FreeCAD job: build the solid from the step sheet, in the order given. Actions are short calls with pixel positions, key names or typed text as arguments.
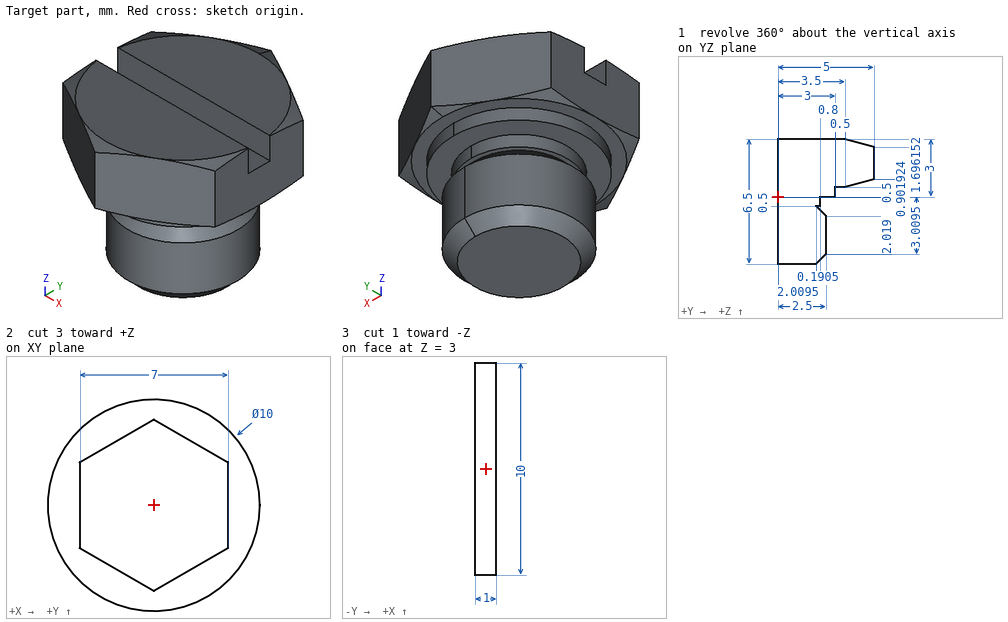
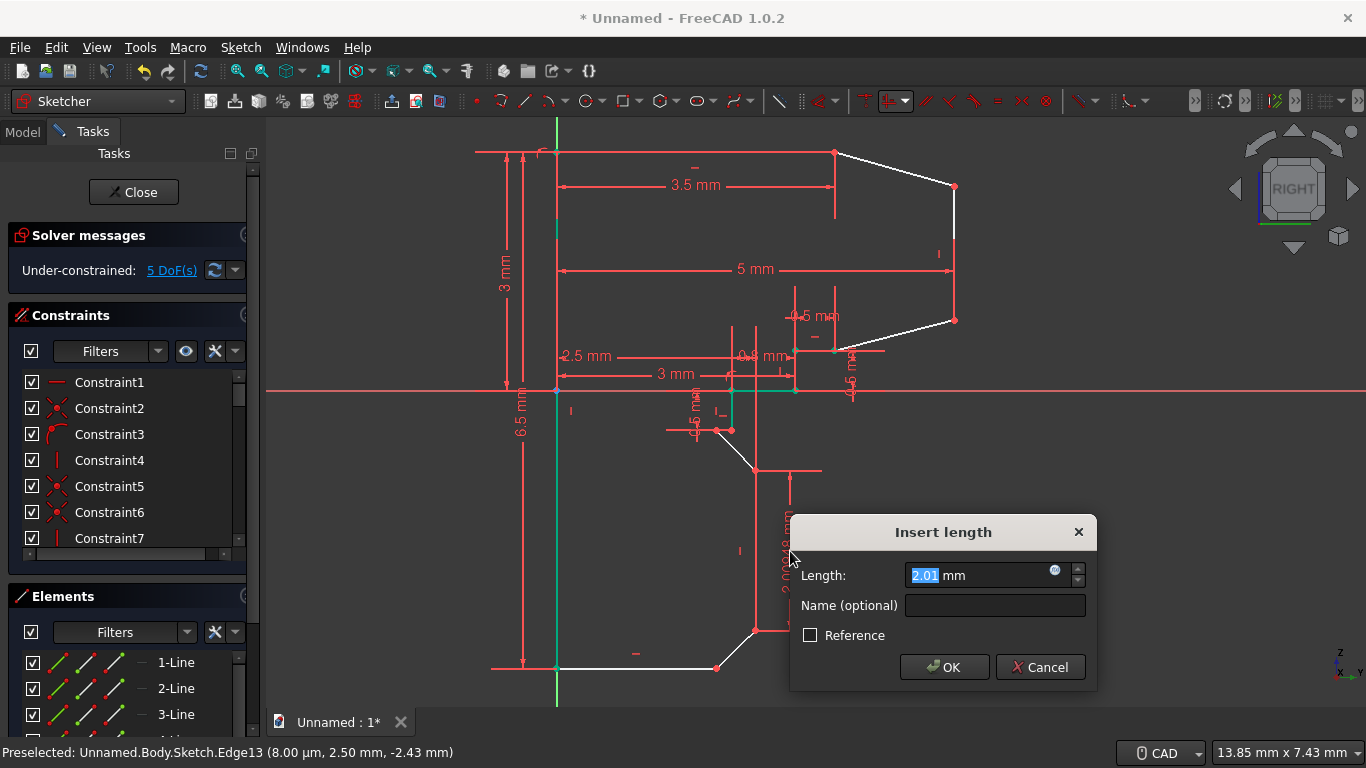
text(2.019)
key(Return)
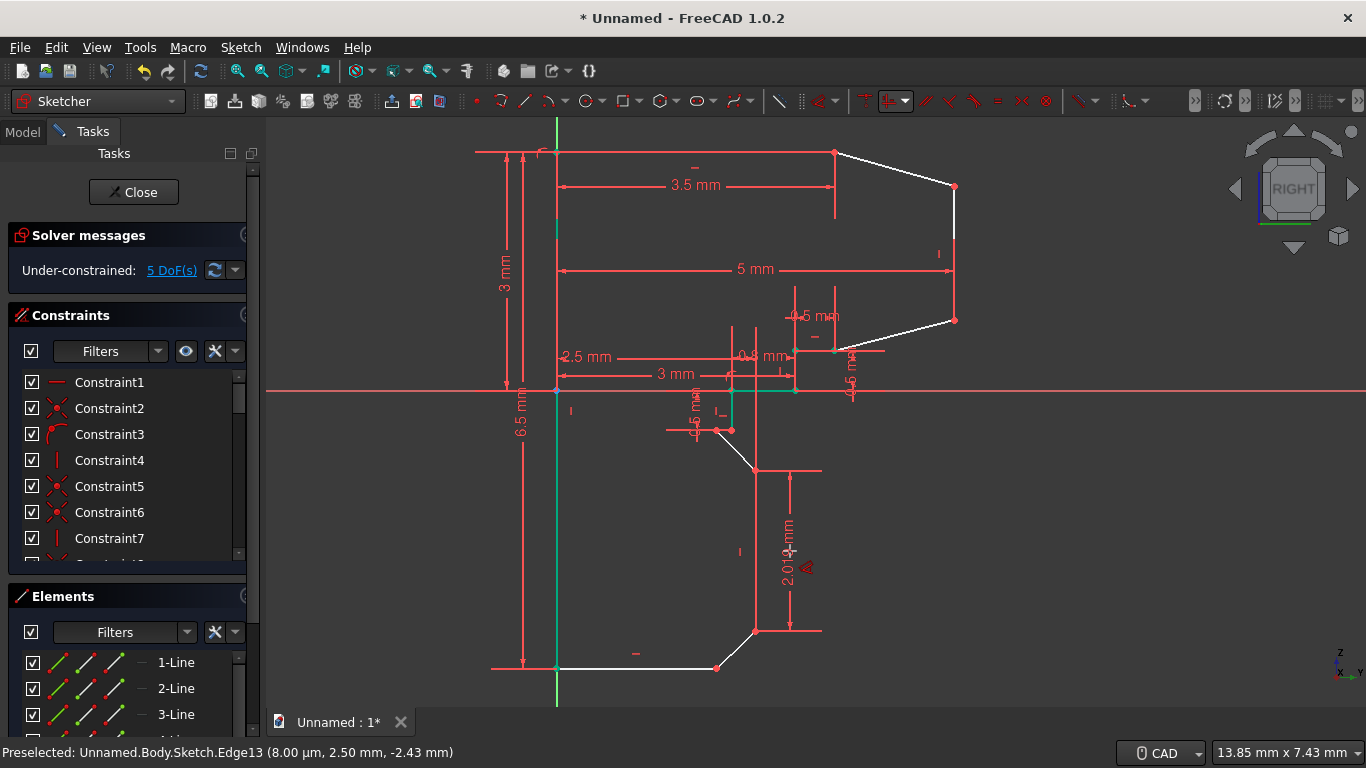
scroll(726, 430, up, 5)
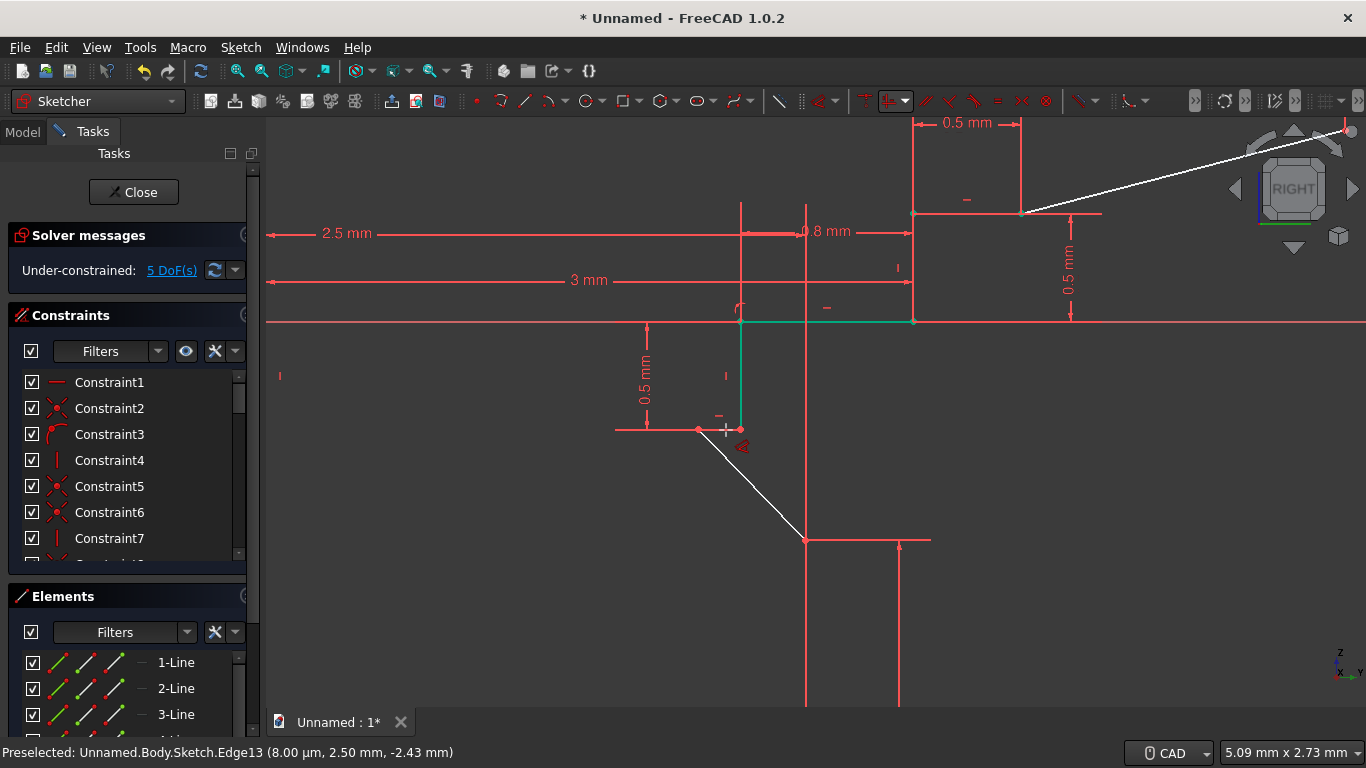
click(724, 430)
click(710, 464)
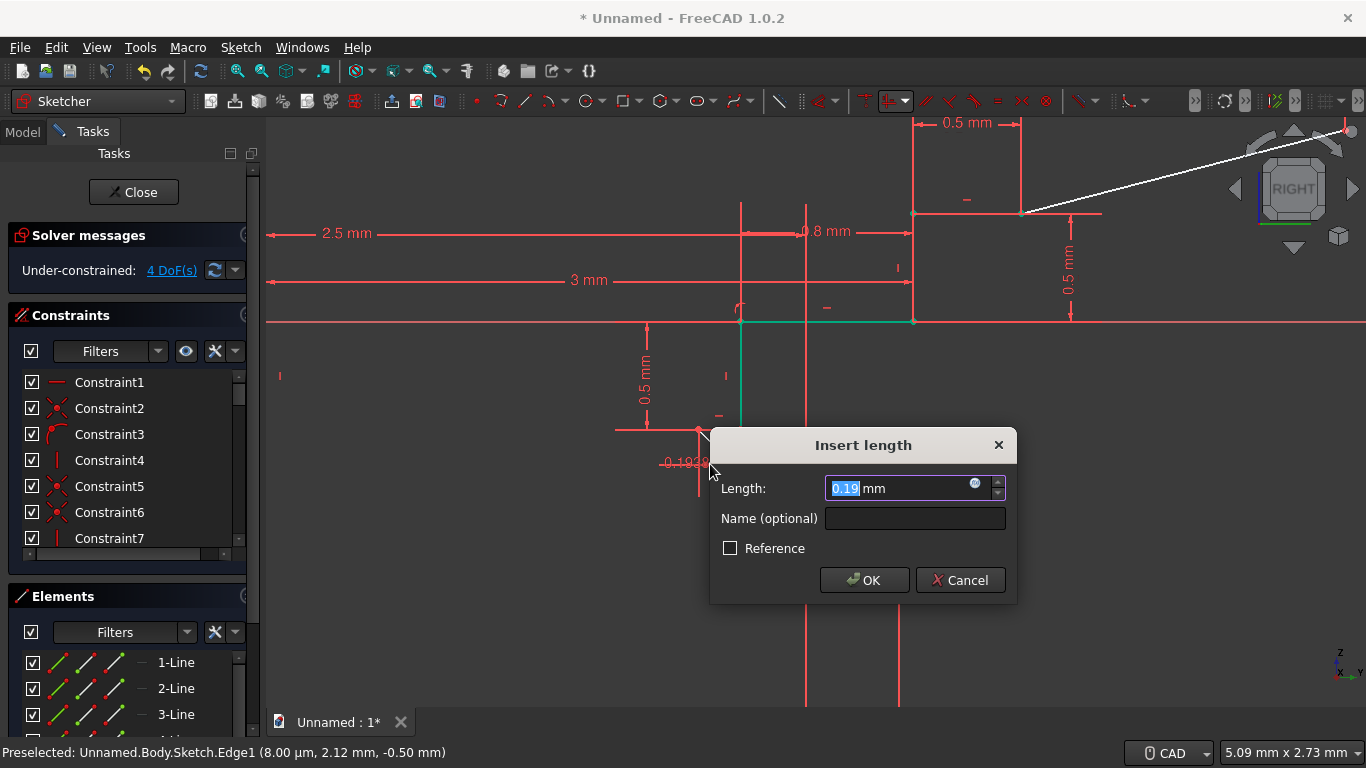
text(0.1905)
key(Return)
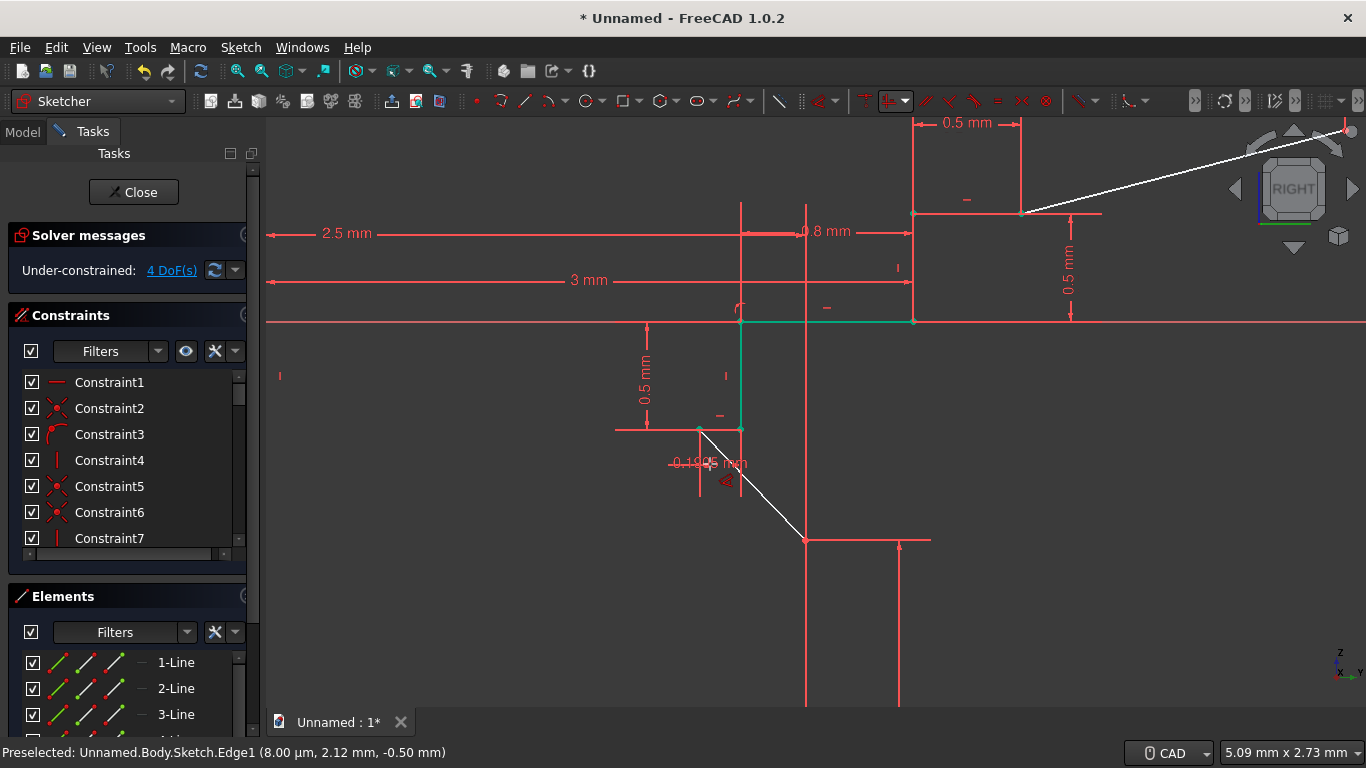
scroll(729, 424, down, 7)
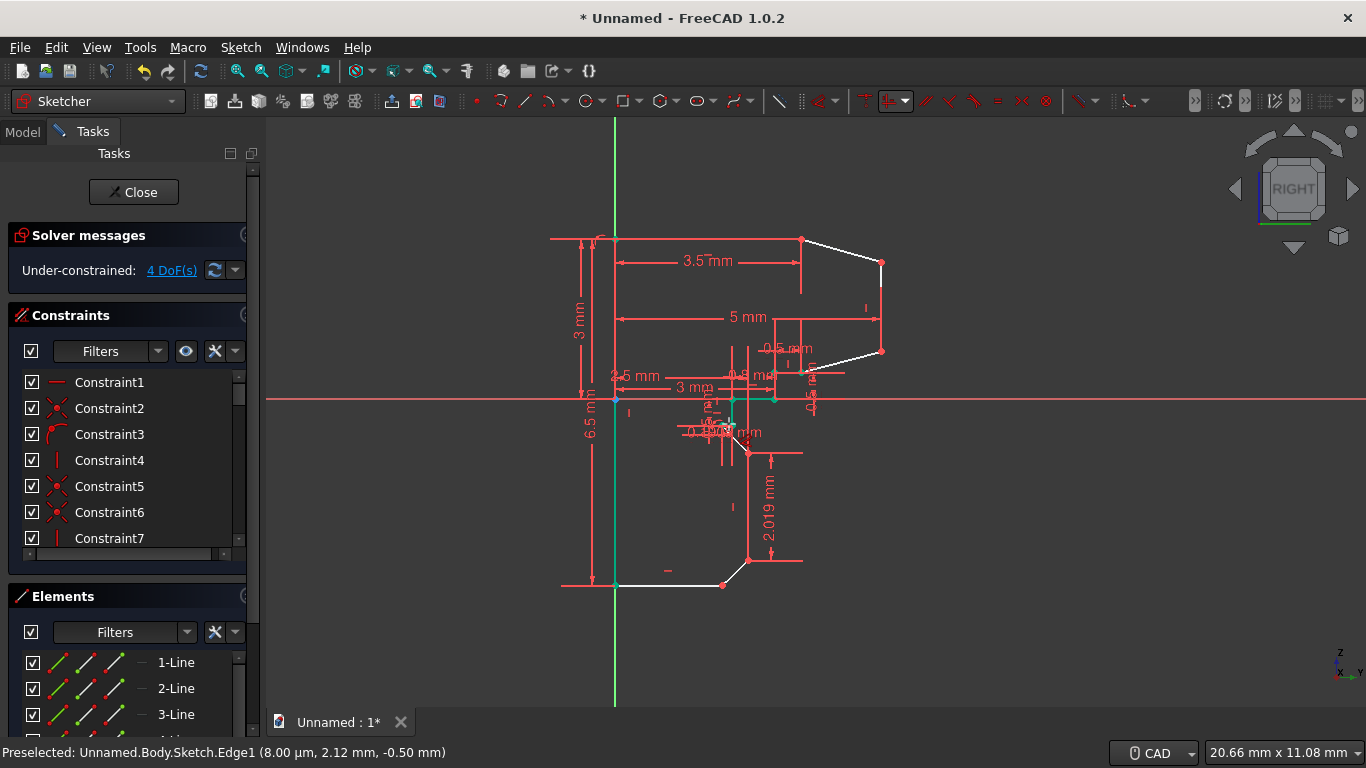
click(647, 586)
click(669, 620)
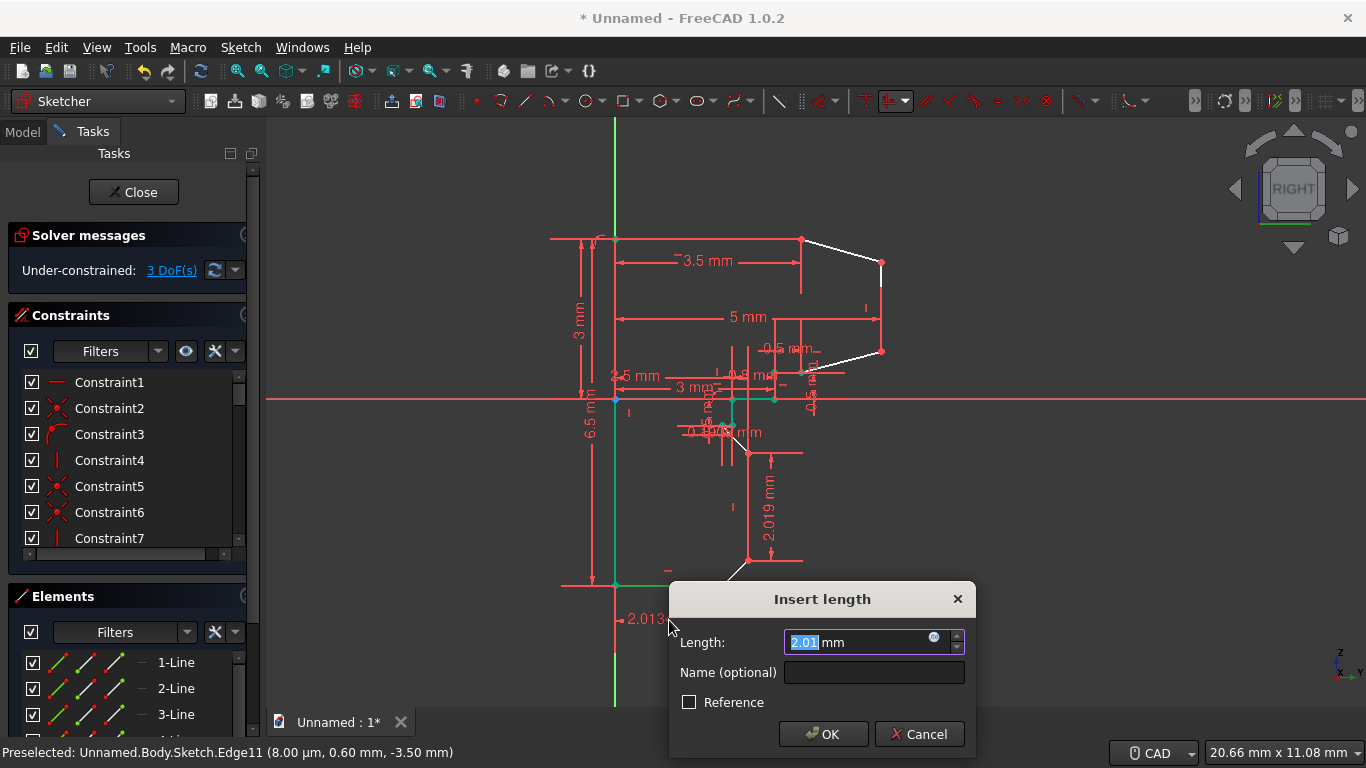
text(2.0095)
key(Return)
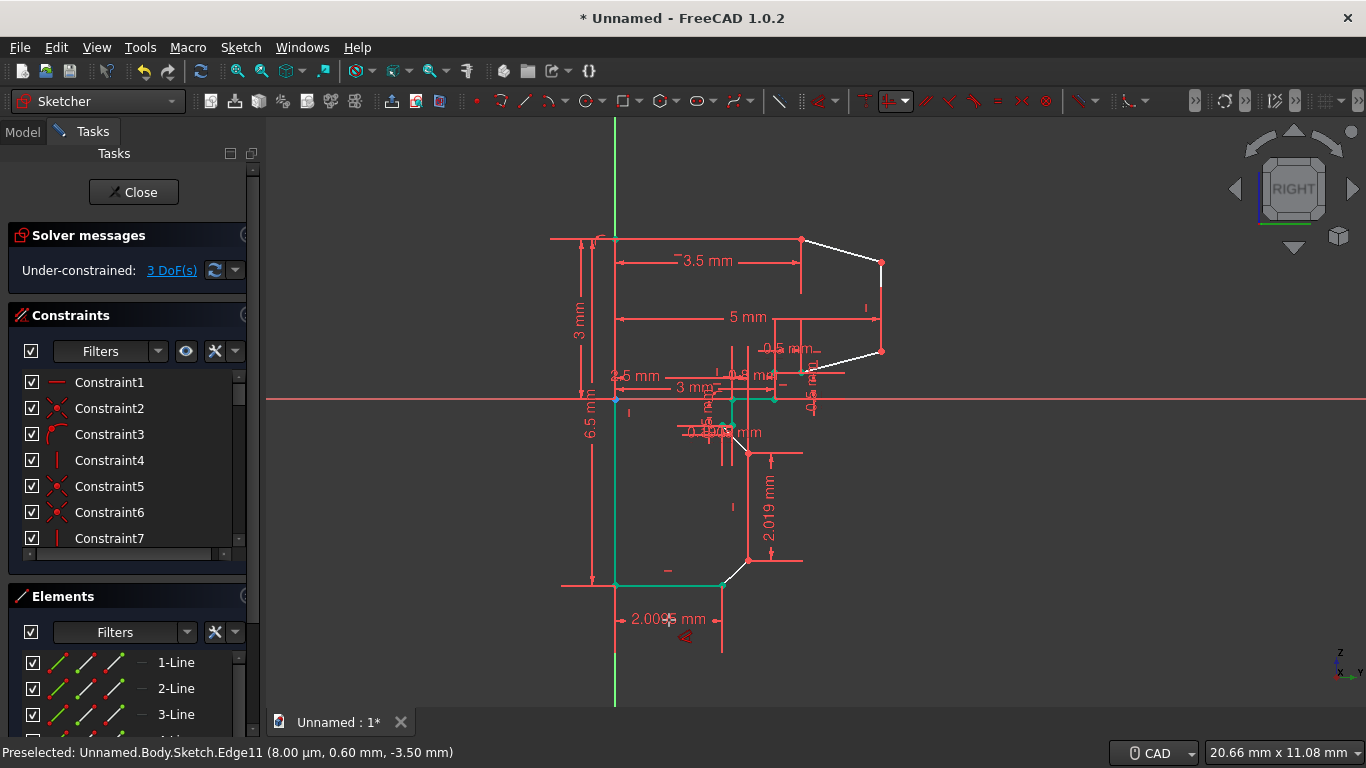
click(748, 561)
click(581, 480)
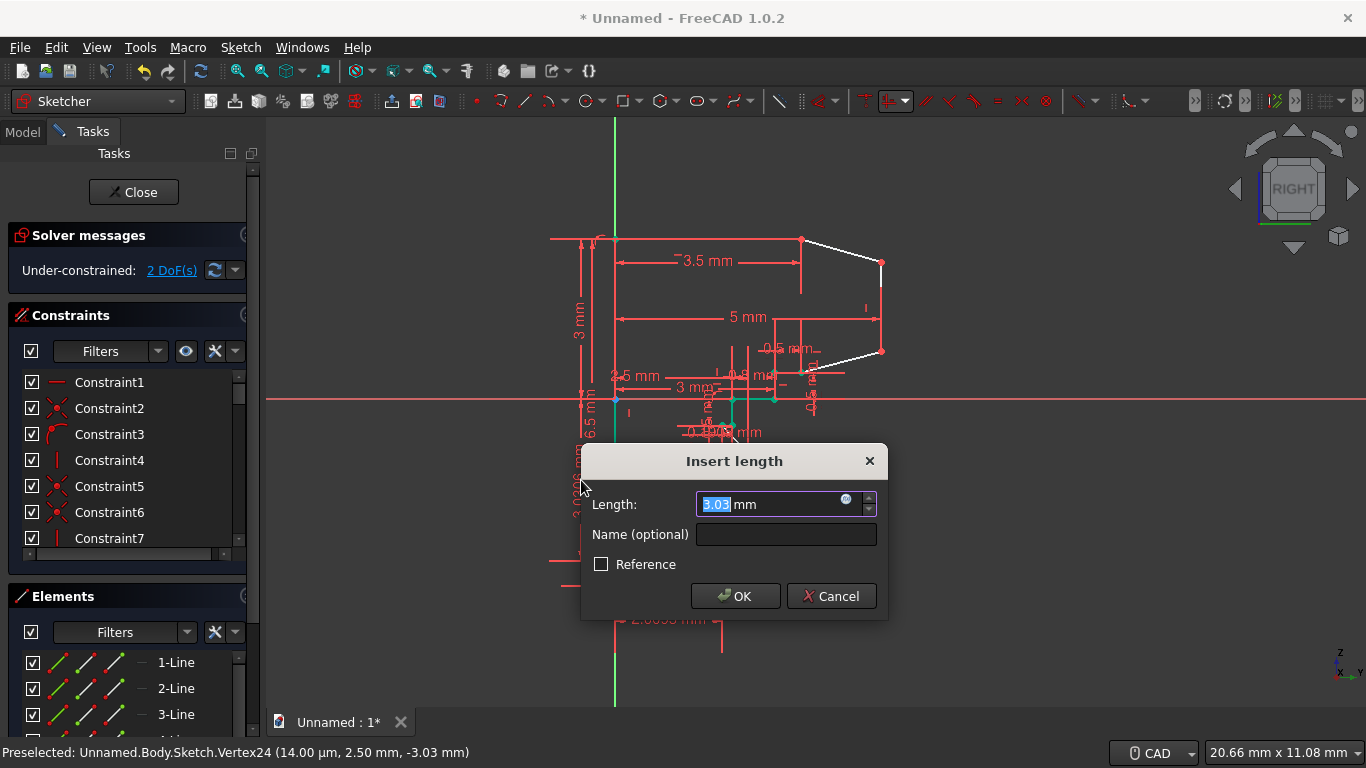
text(3.0095)
key(Return)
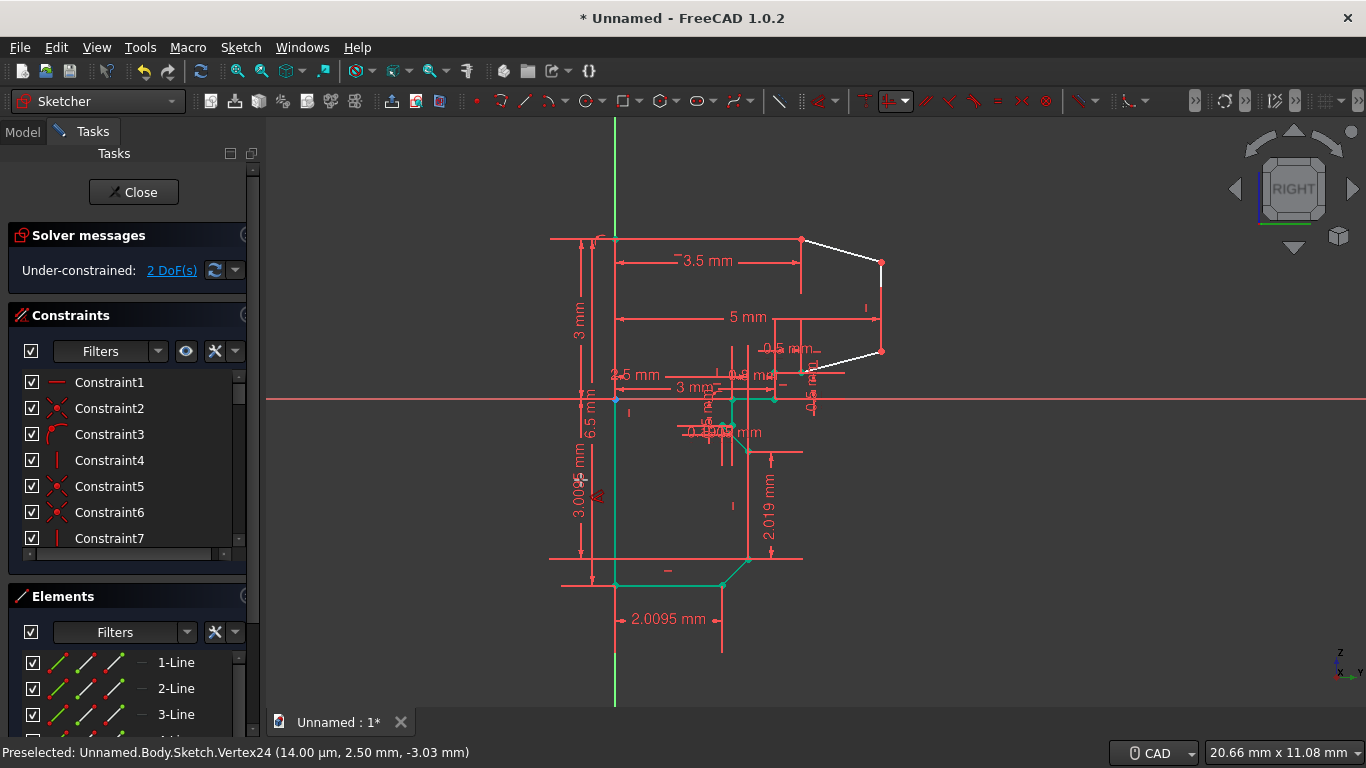
click(881, 325)
click(915, 307)